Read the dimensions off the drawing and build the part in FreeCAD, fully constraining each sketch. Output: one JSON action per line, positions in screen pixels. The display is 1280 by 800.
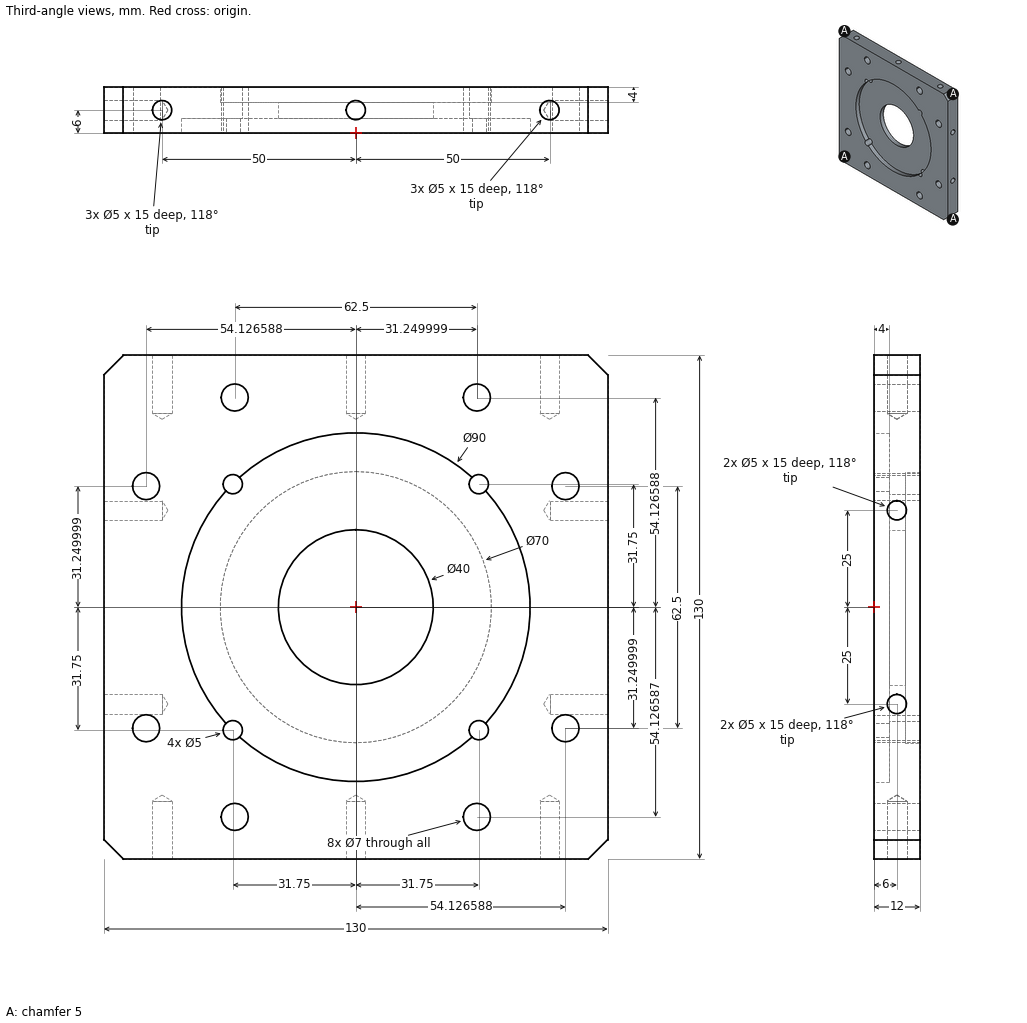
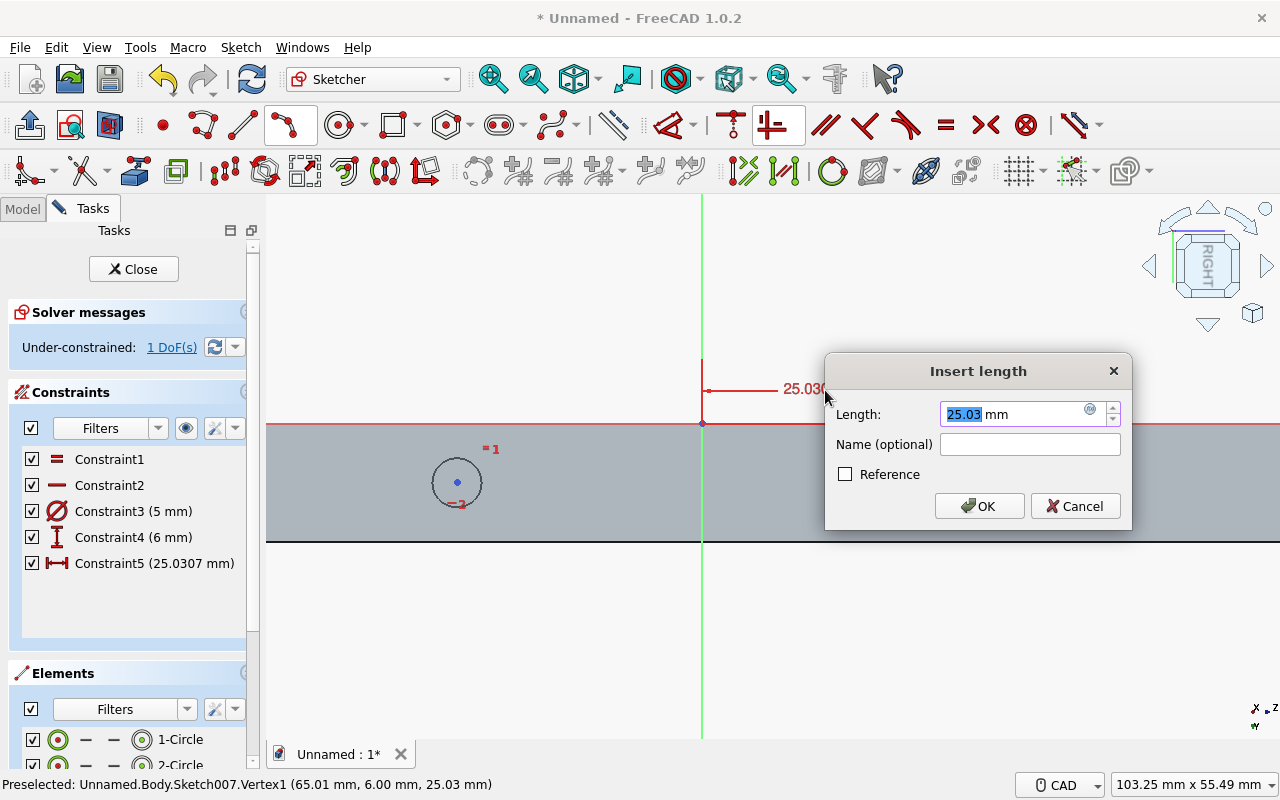
{"action": "type", "text": "25"}
{"action": "key", "text": "Return"}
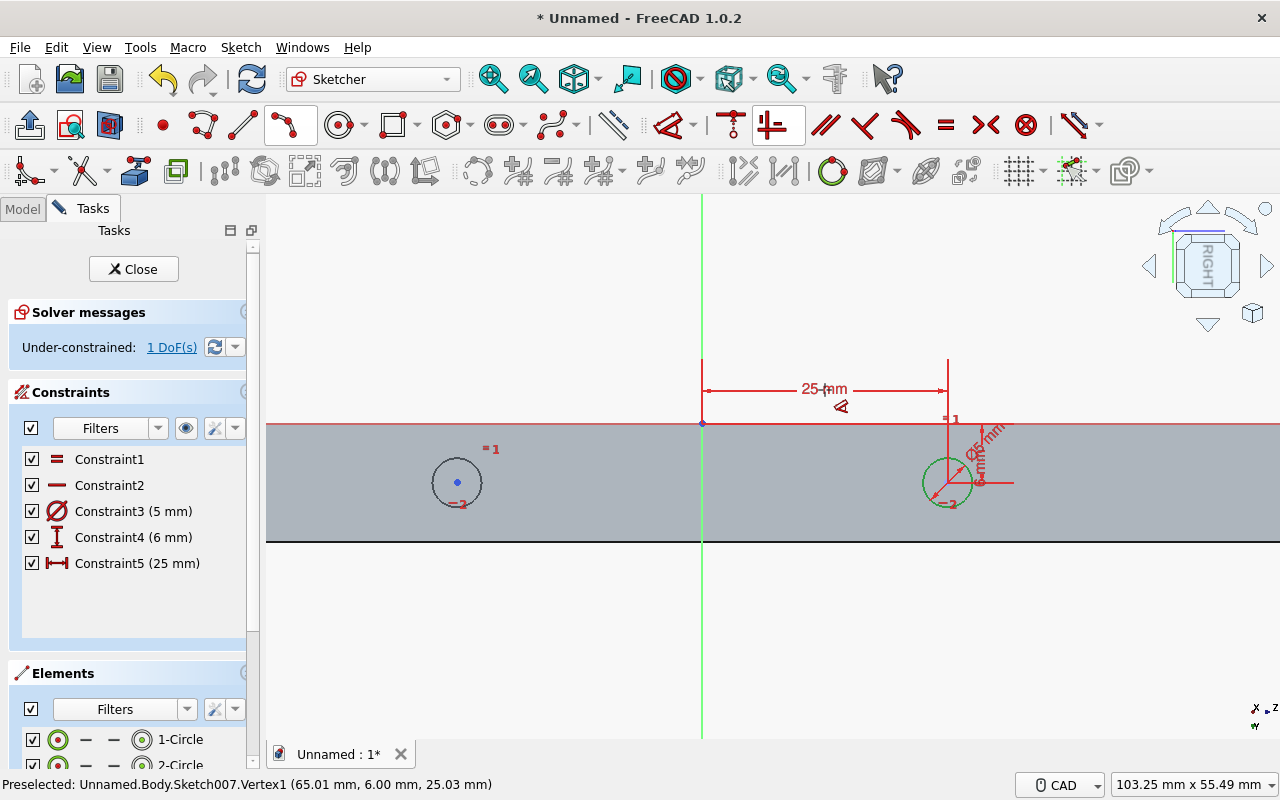
{"action": "left_click", "coordinate": [457, 483]}
{"action": "left_click", "coordinate": [580, 390]}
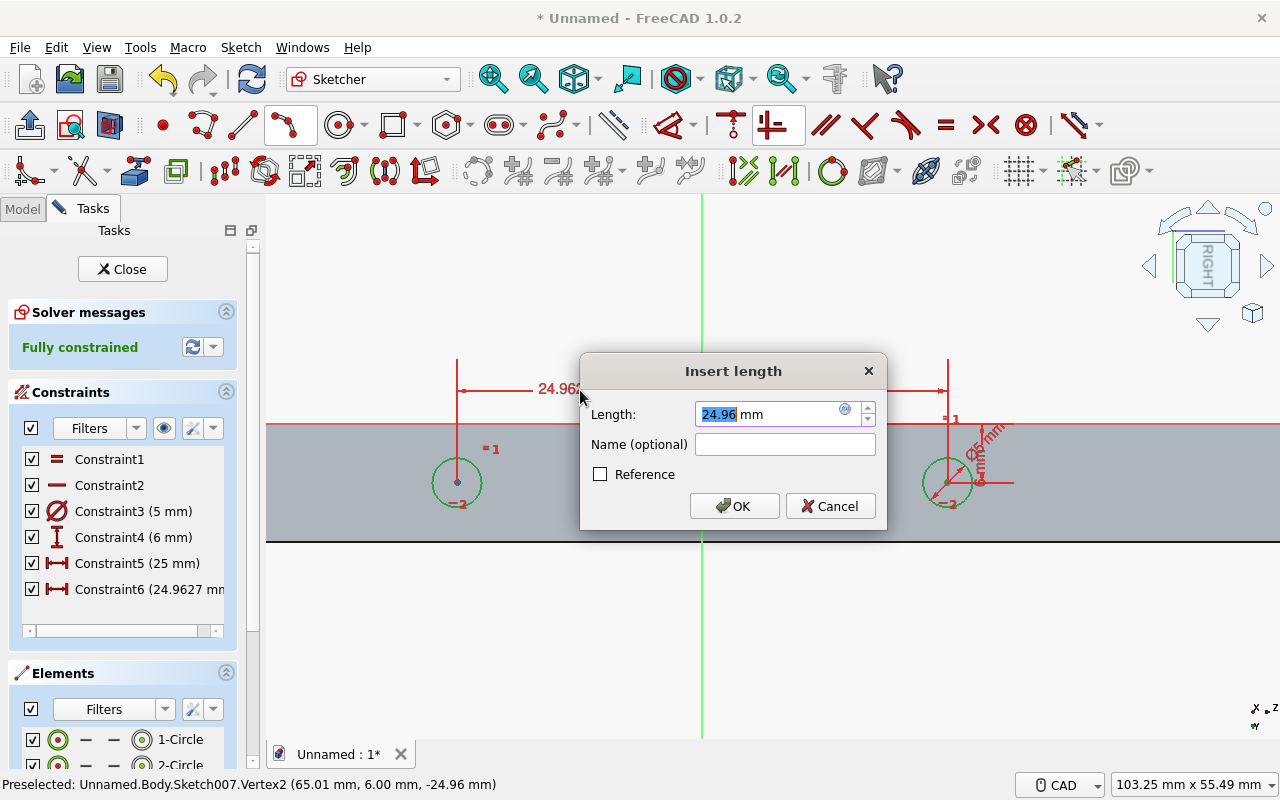
{"action": "type", "text": "25"}
{"action": "key", "text": "Return"}
{"action": "key", "text": "Escape"}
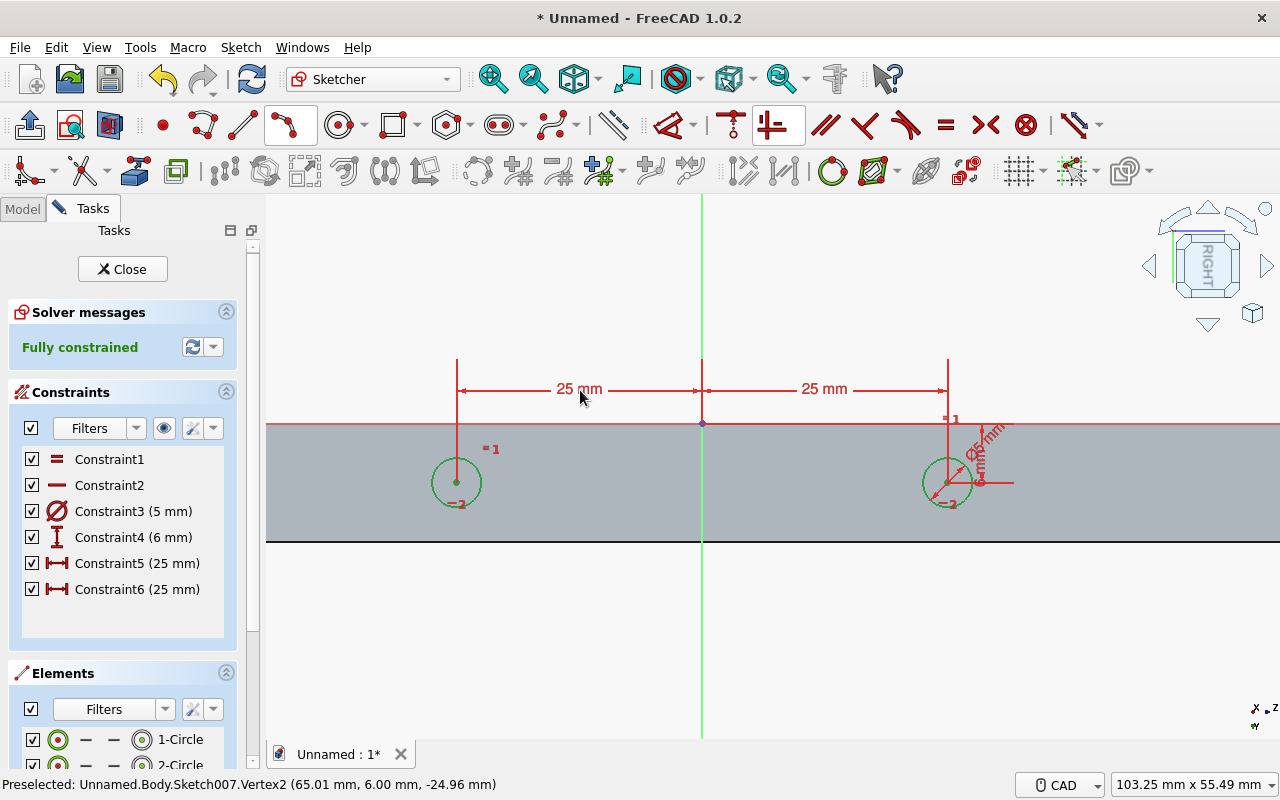
{"action": "left_click", "coordinate": [123, 269]}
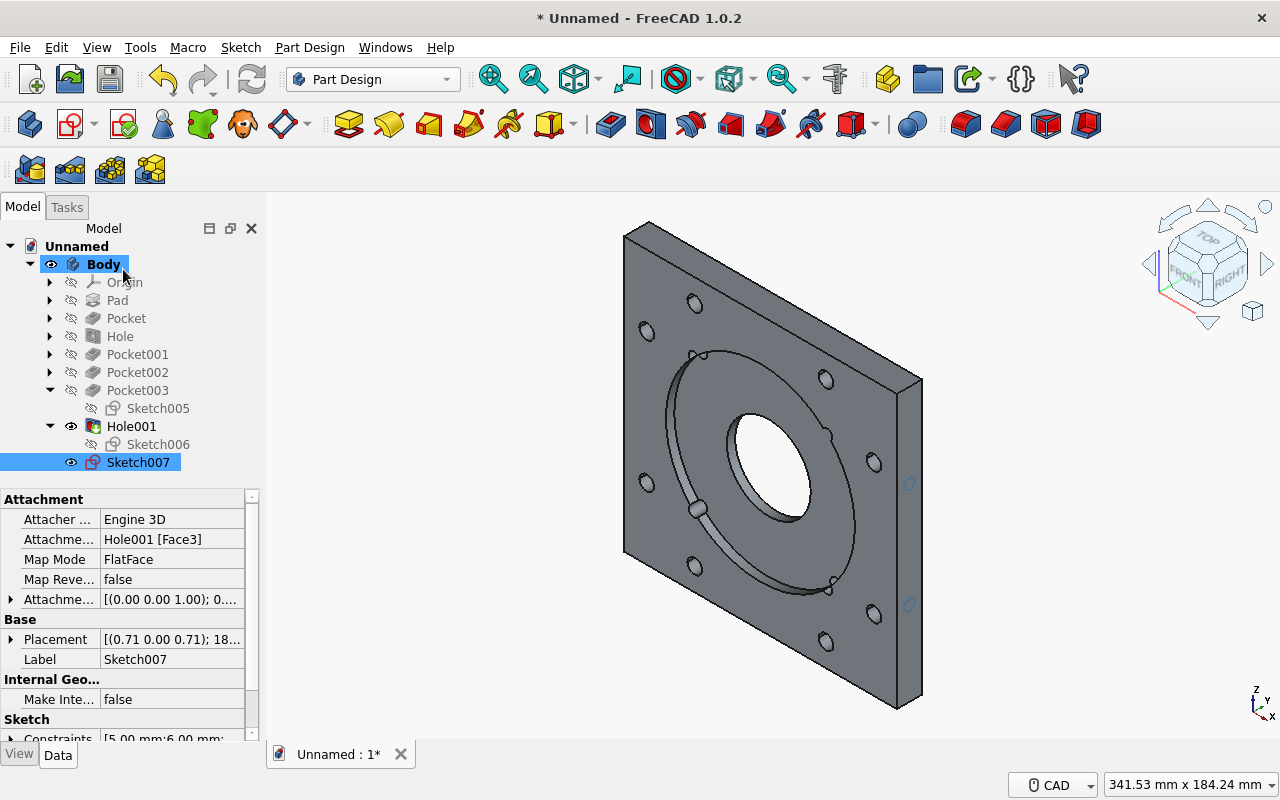
{"action": "left_click", "coordinate": [652, 124]}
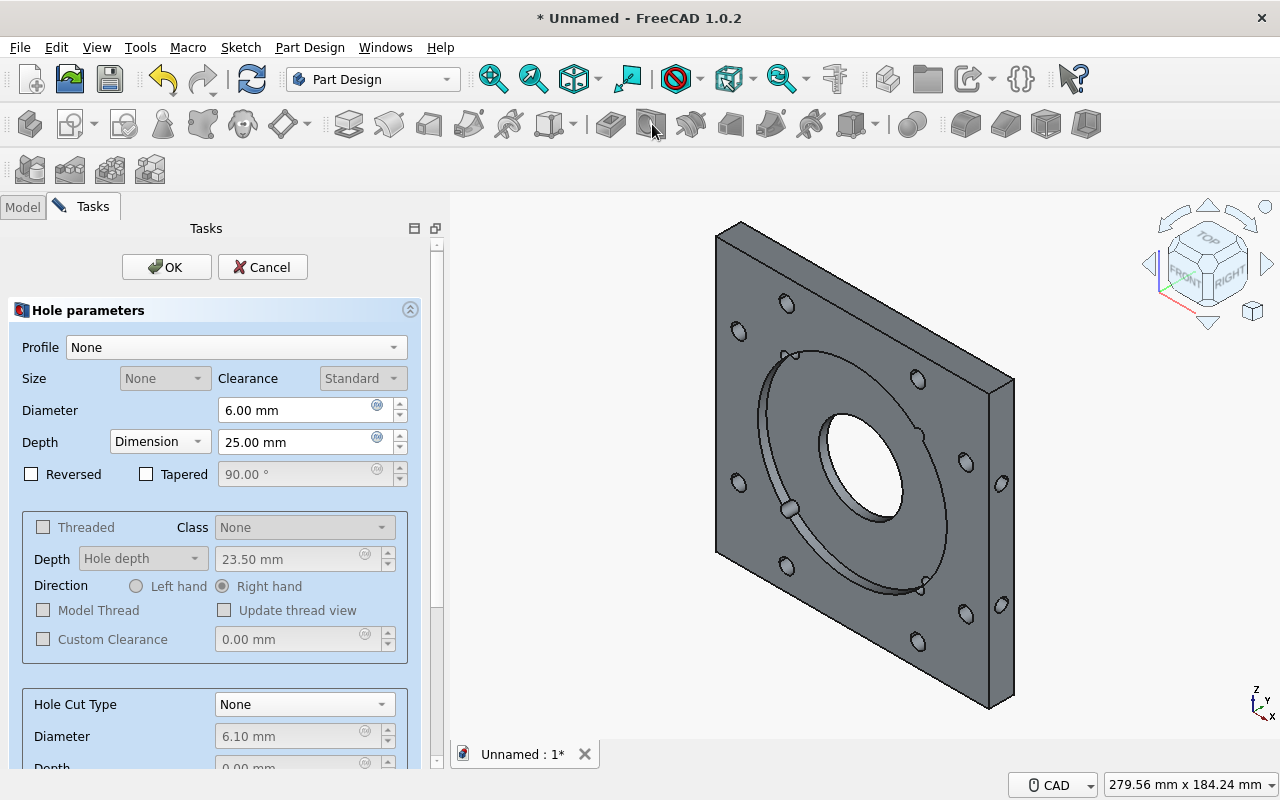
{"action": "triple_click", "coordinate": [305, 410]}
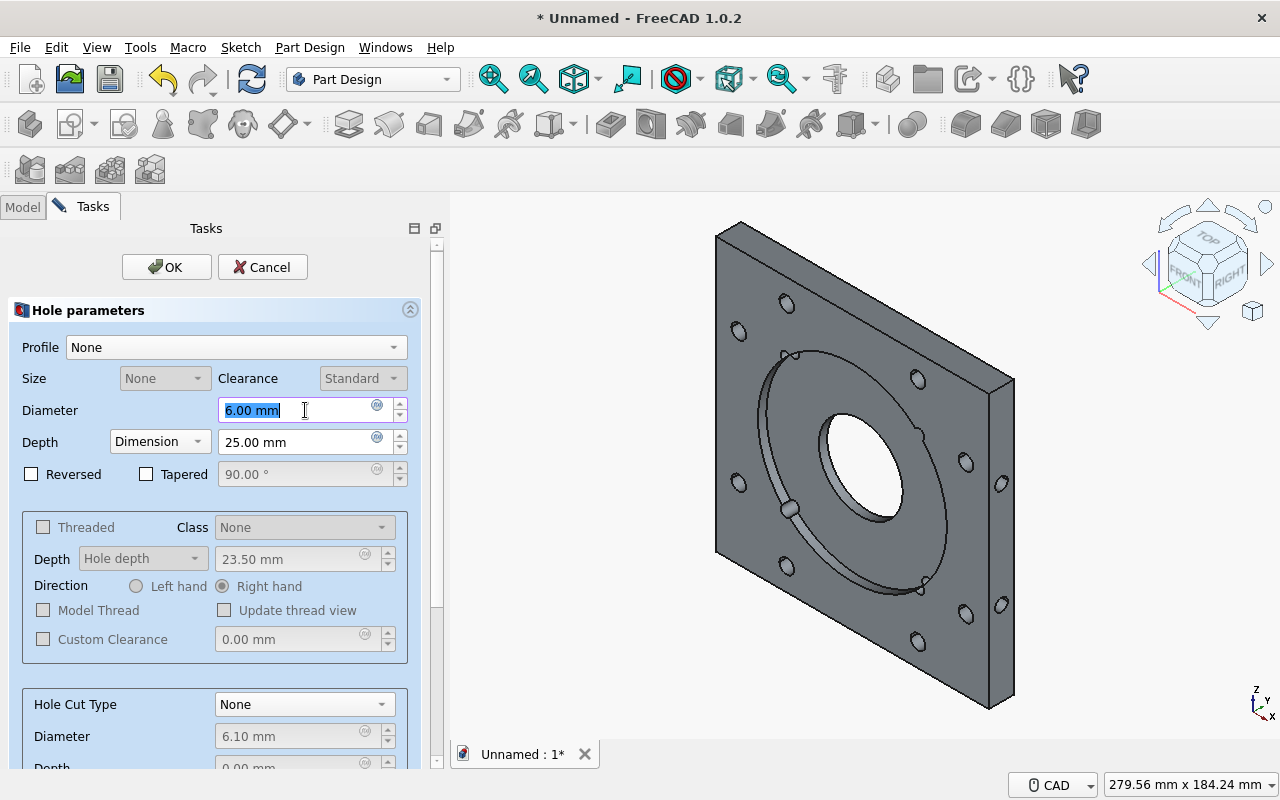
{"action": "type", "text": "5"}
{"action": "key", "text": "Tab"}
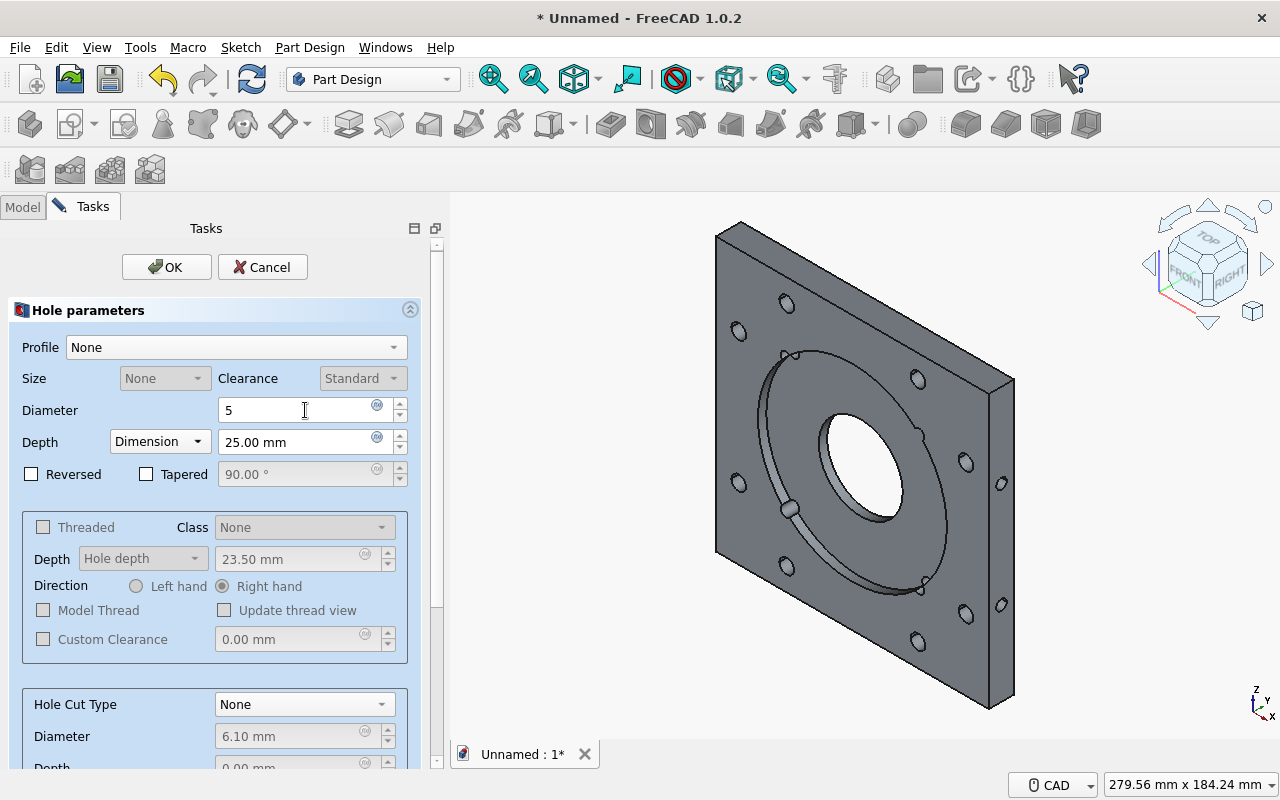
{"action": "triple_click", "coordinate": [305, 442]}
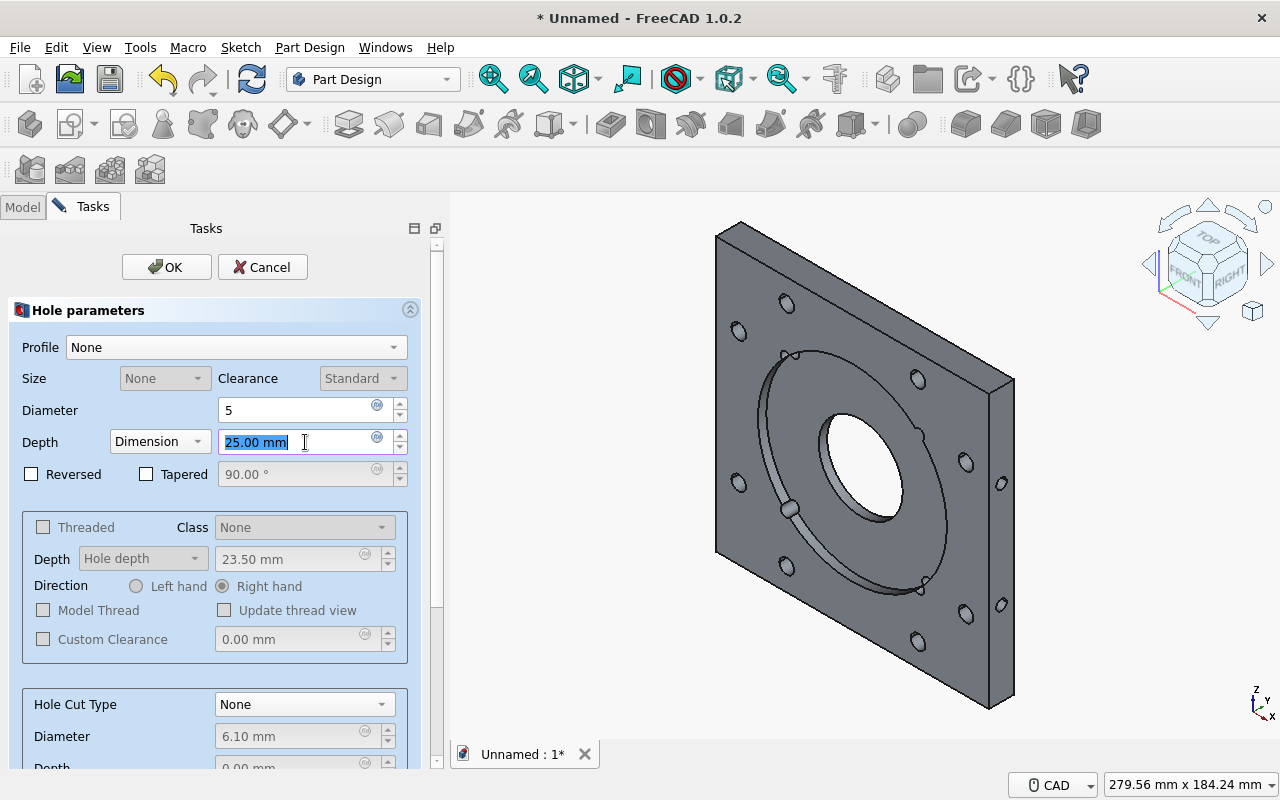
{"action": "type", "text": "15"}
{"action": "key", "text": "Tab"}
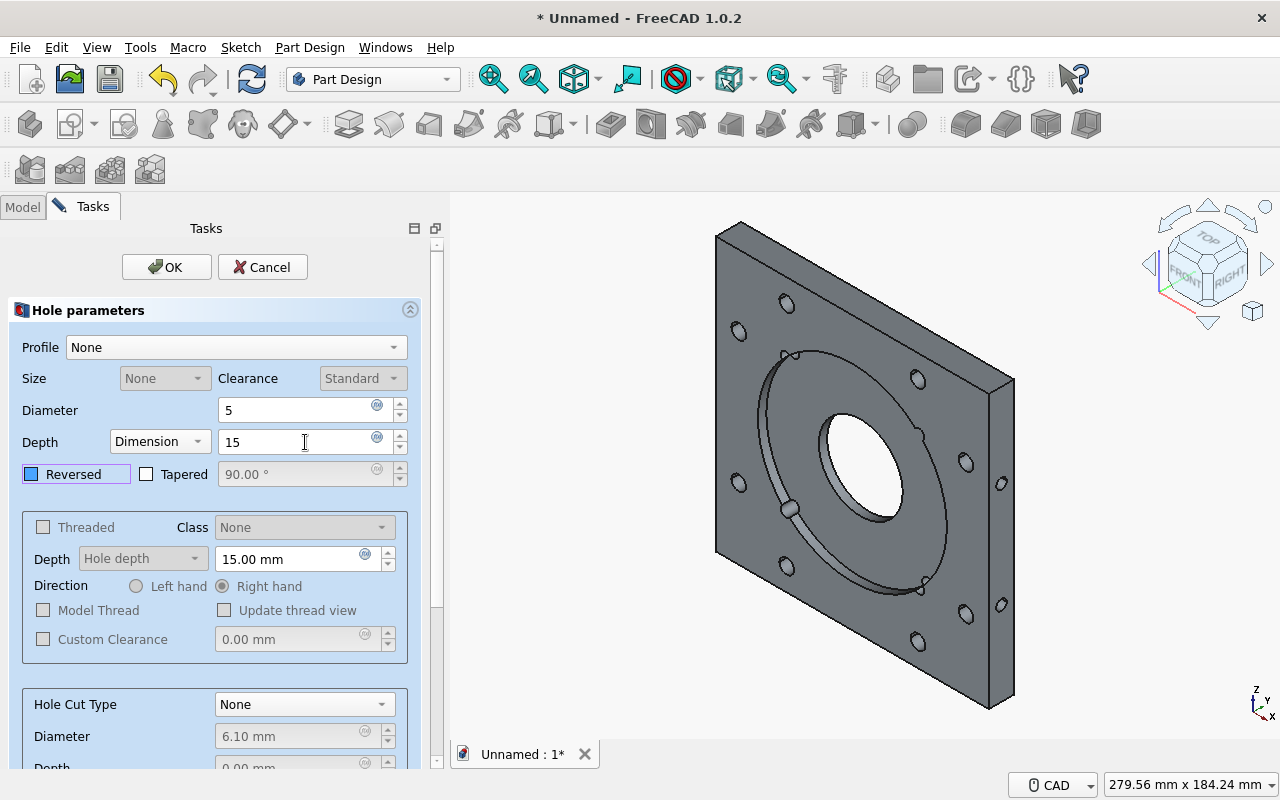
{"action": "left_click", "coordinate": [167, 267]}